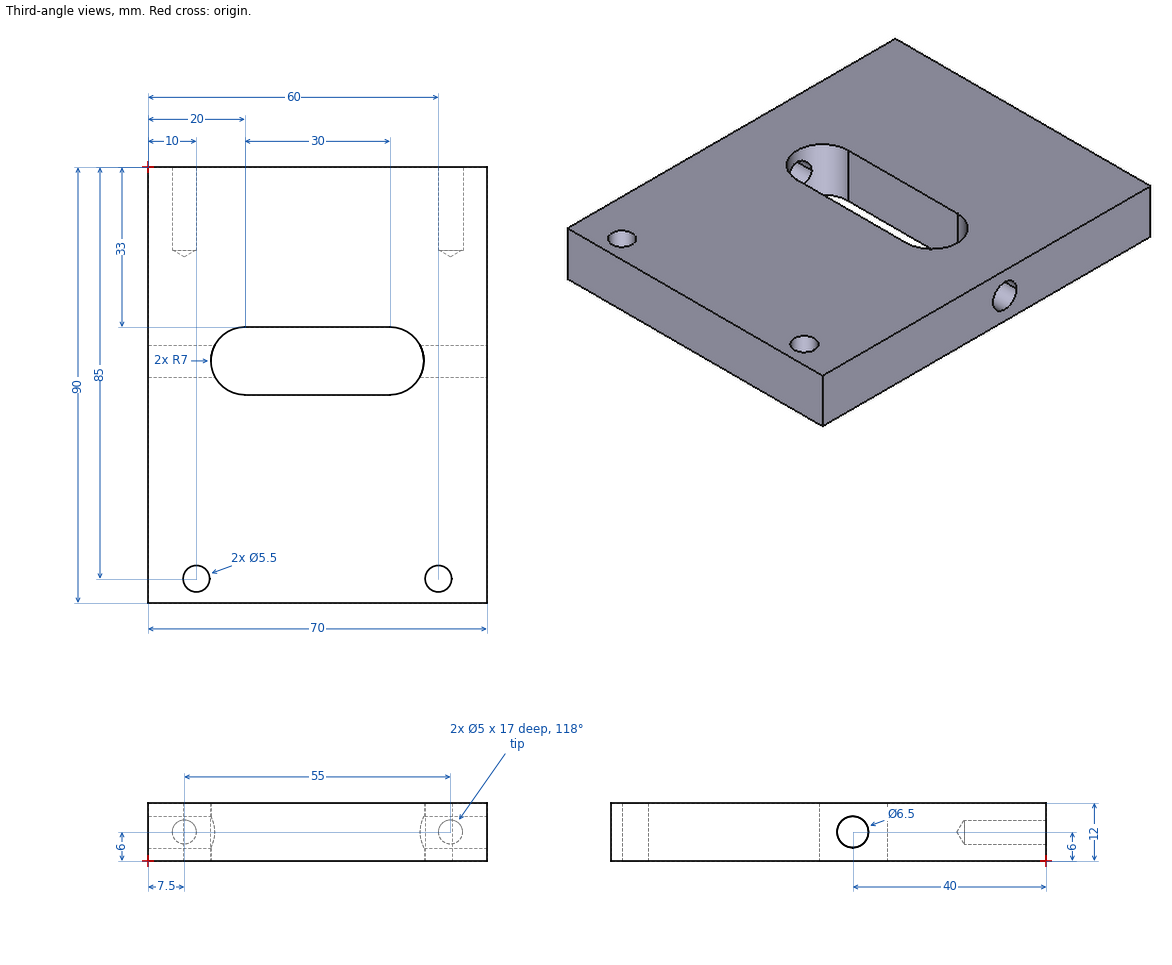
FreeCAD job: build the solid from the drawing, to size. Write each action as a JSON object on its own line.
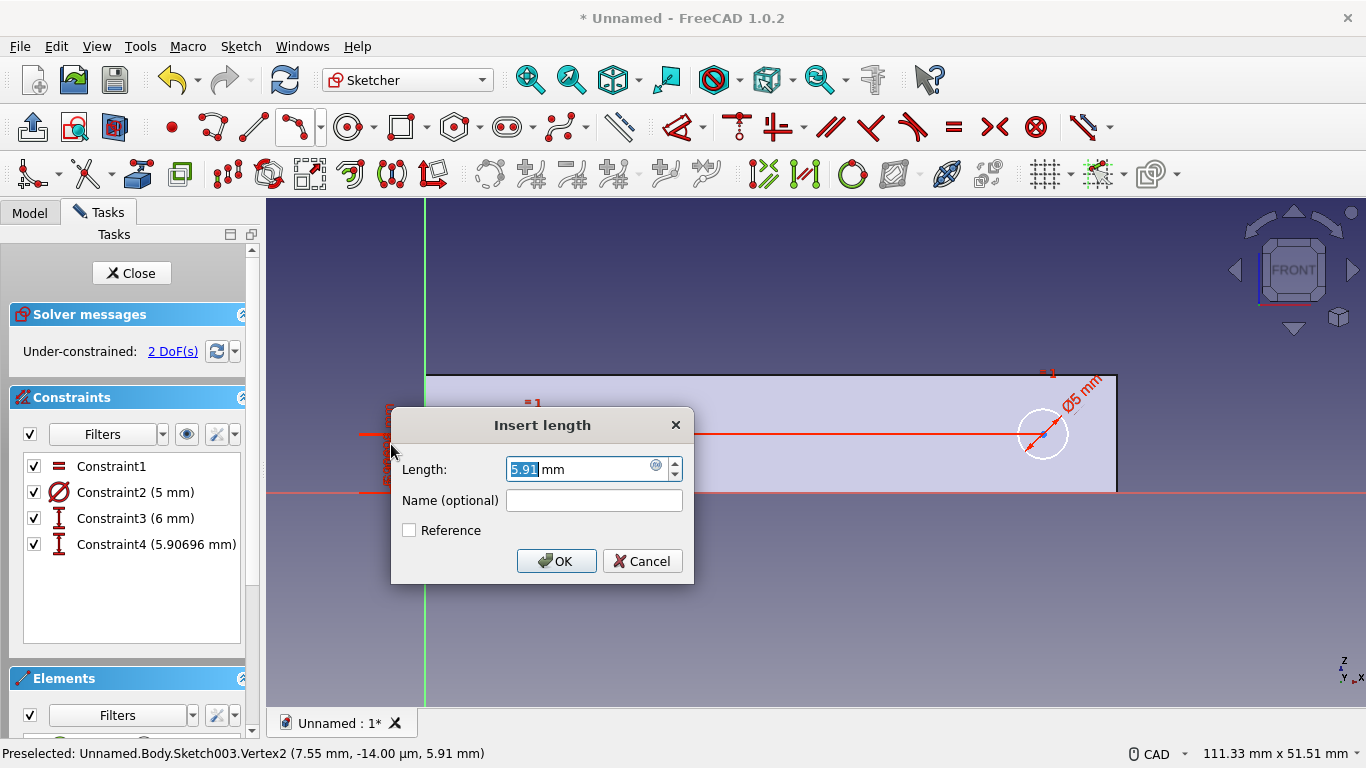
{"action": "type", "text": "6"}
{"action": "key", "text": "Return"}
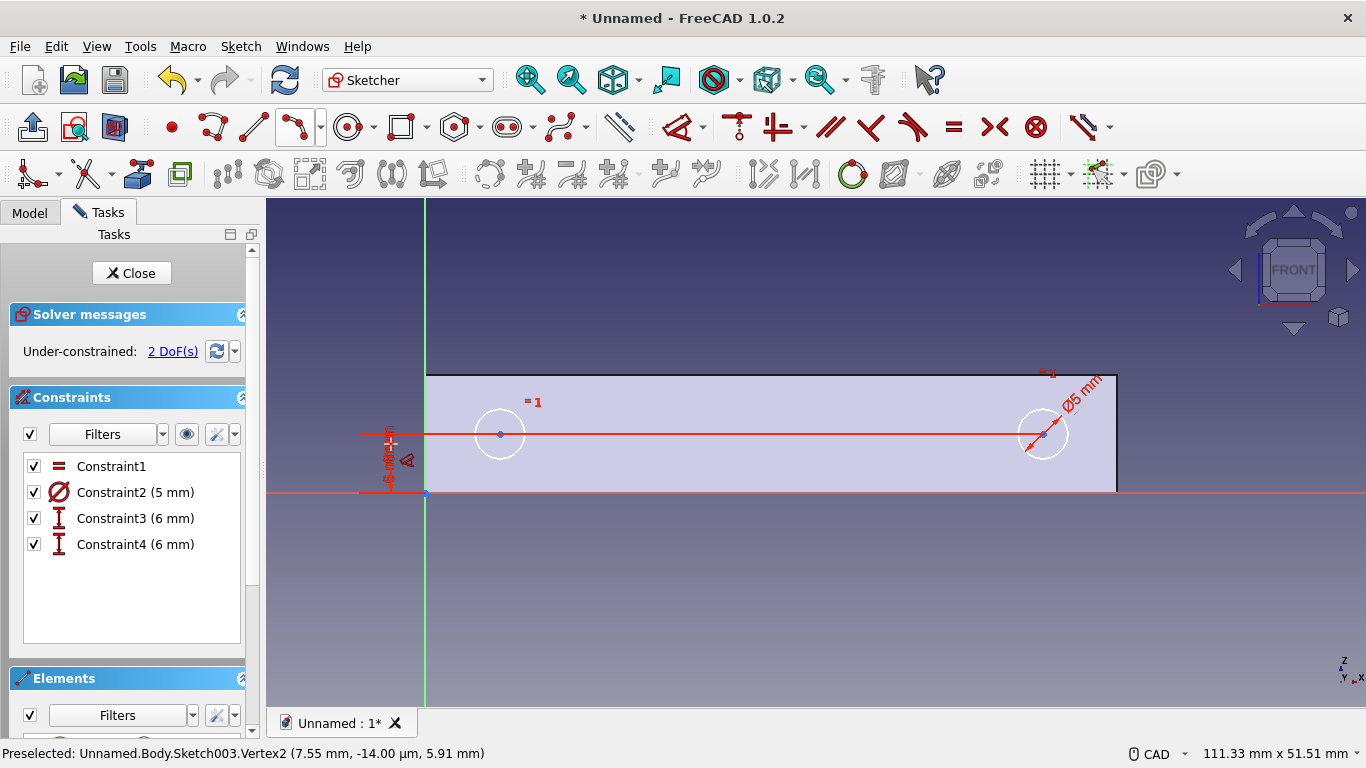
{"action": "left_click", "coordinate": [500, 434]}
{"action": "left_click", "coordinate": [463, 527]}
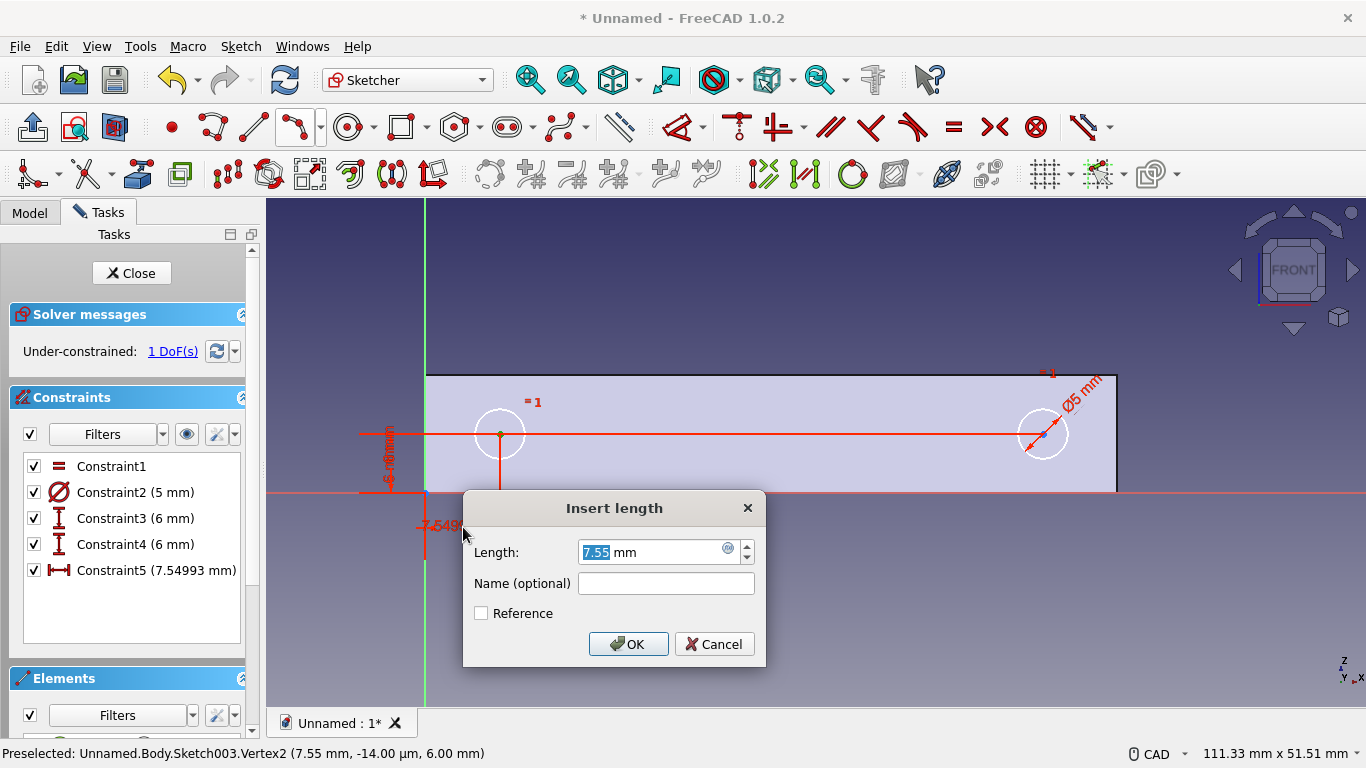
{"action": "type", "text": "7.5"}
{"action": "key", "text": "Return"}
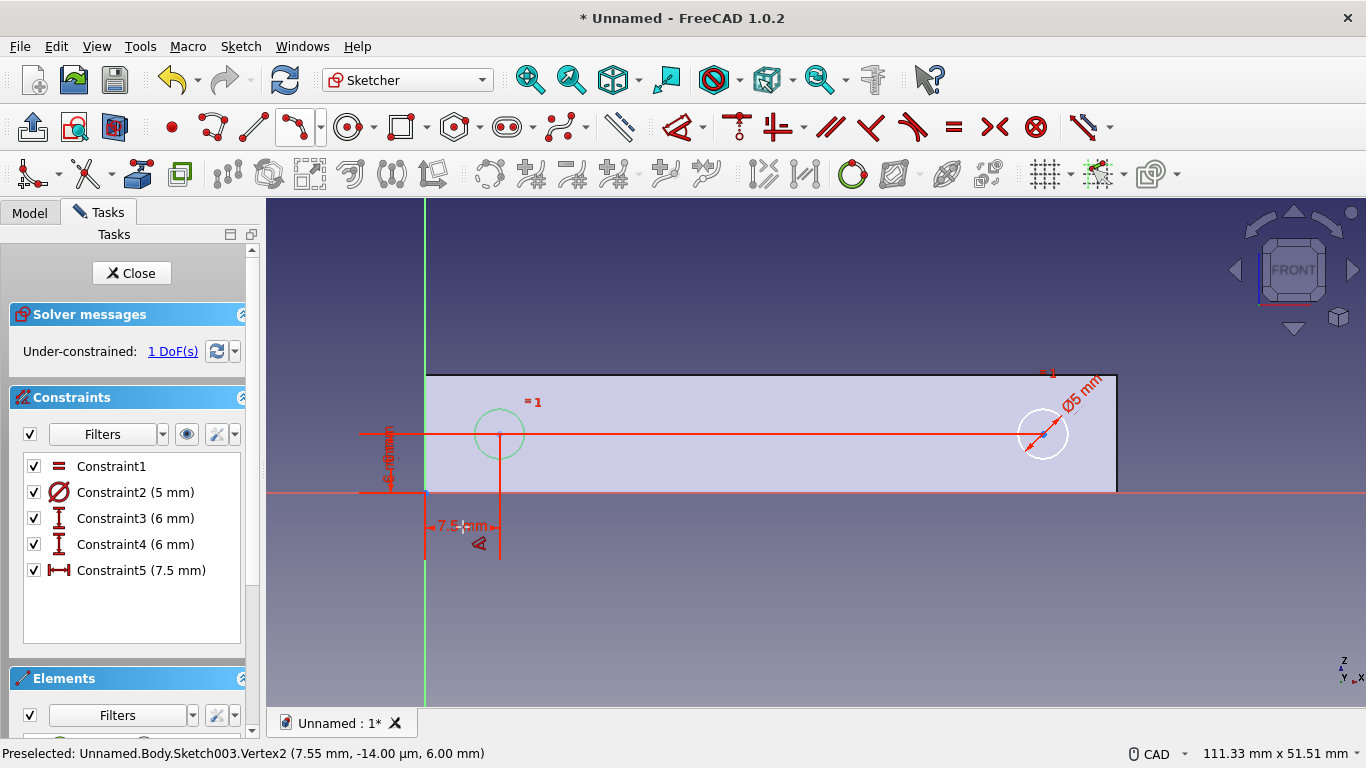
{"action": "left_click", "coordinate": [1043, 434]}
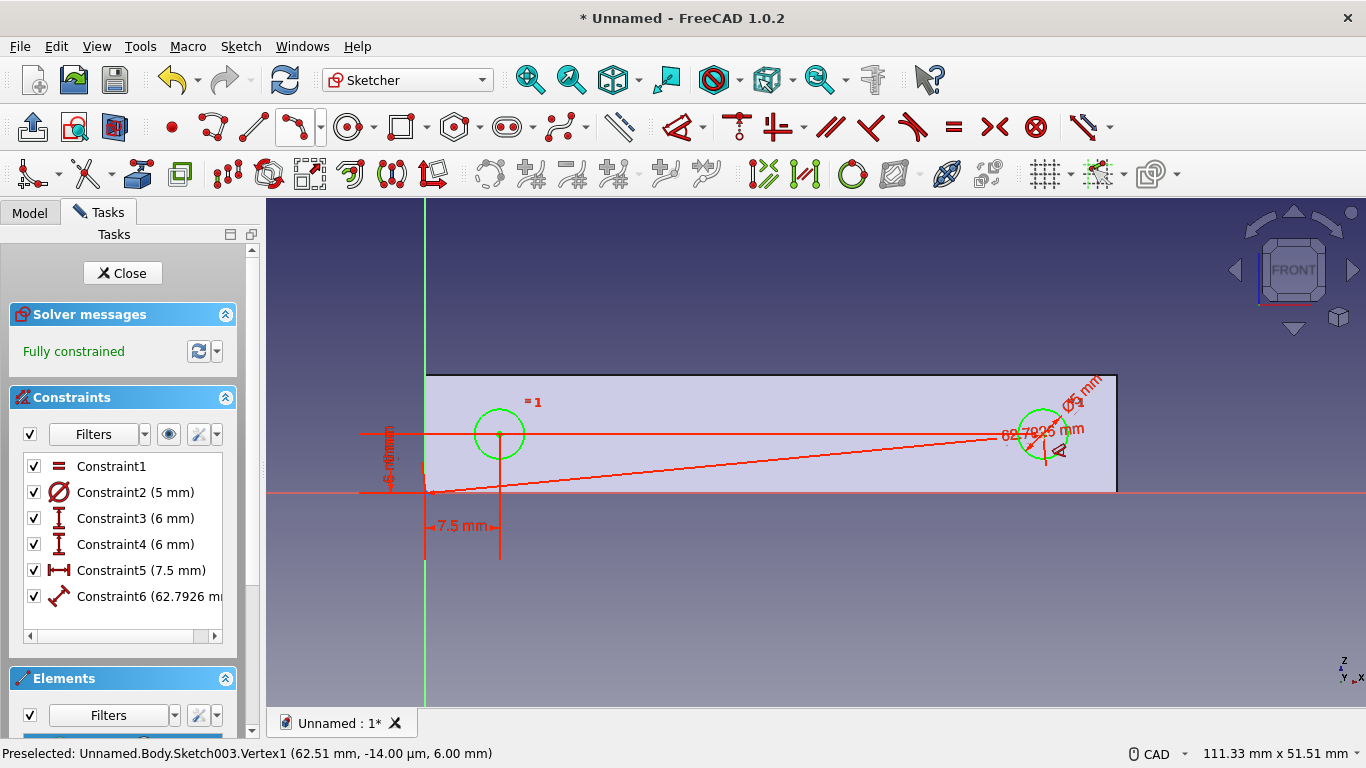
{"action": "left_click", "coordinate": [500, 434]}
{"action": "left_click", "coordinate": [771, 400]}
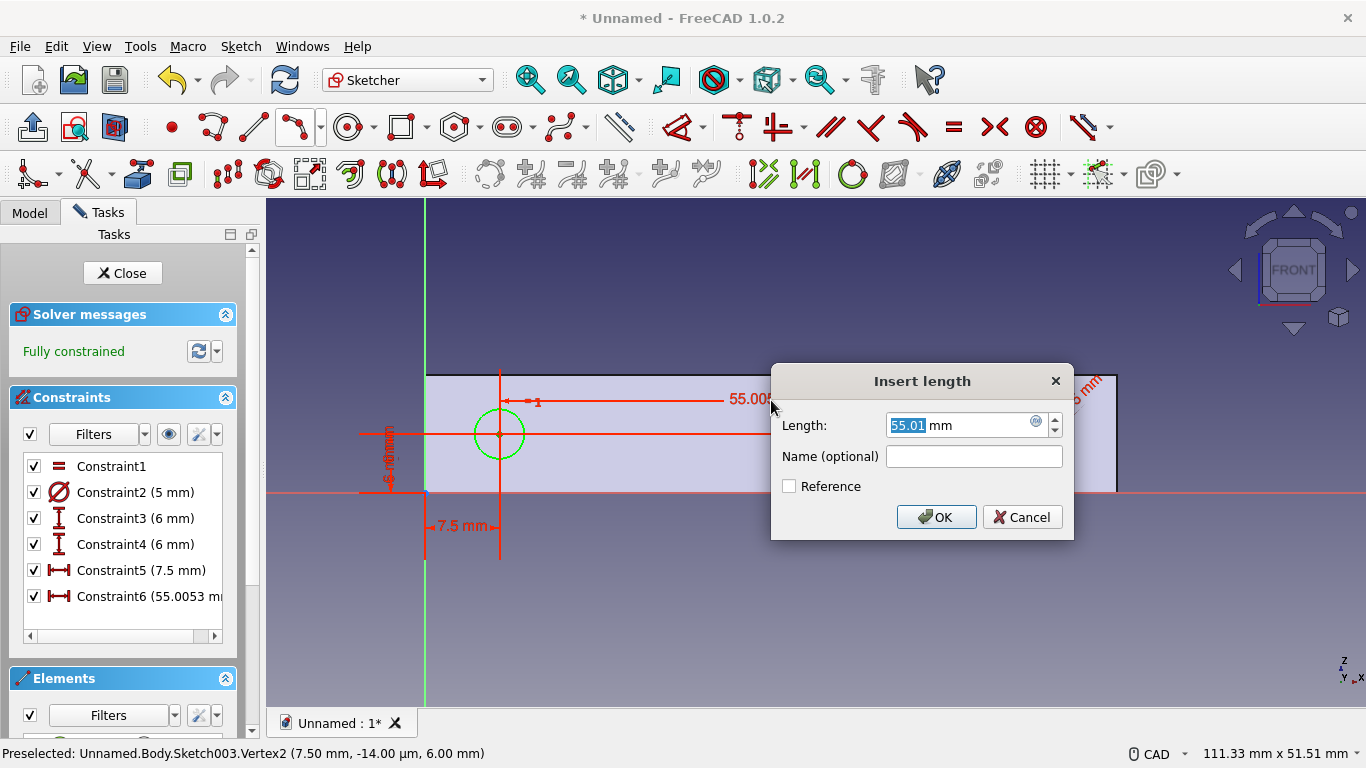
{"action": "type", "text": "55"}
{"action": "key", "text": "Return"}
{"action": "key", "text": "Escape"}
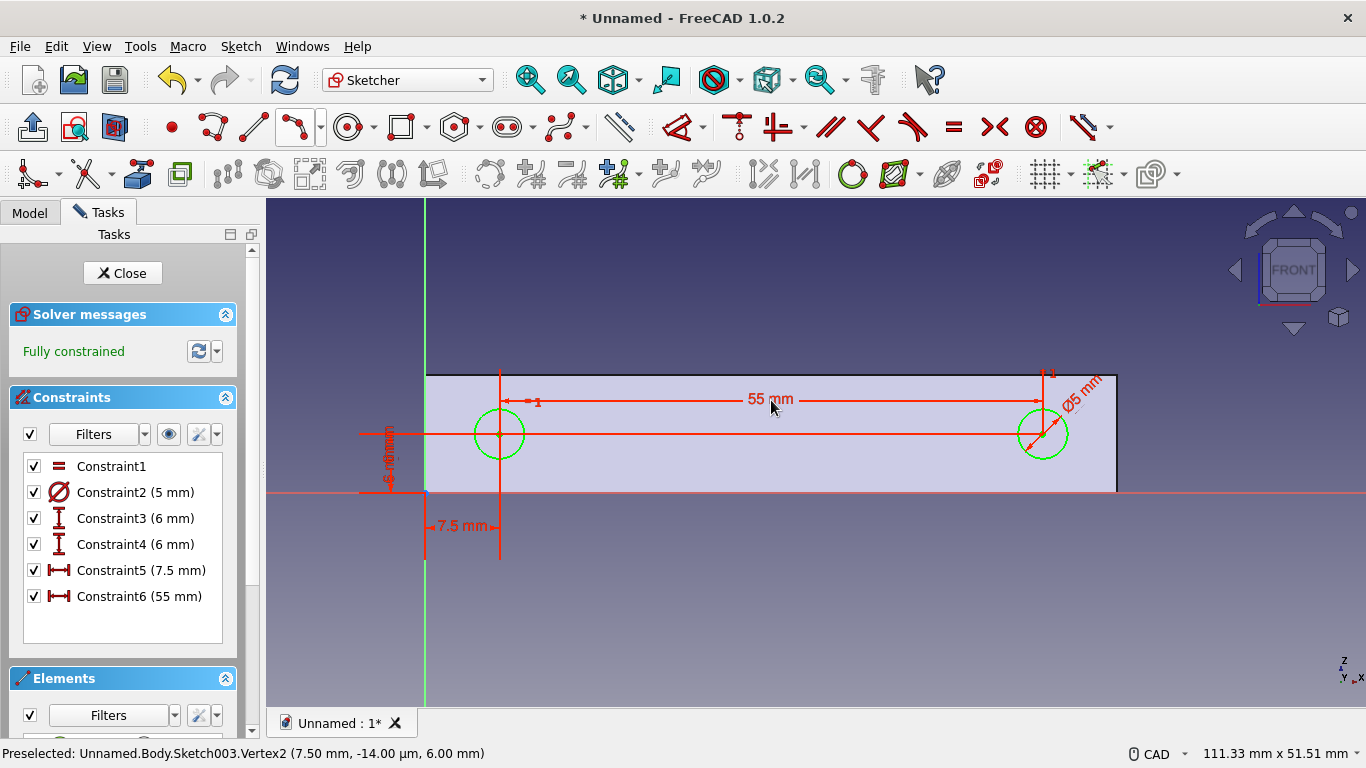
{"action": "left_click", "coordinate": [123, 273]}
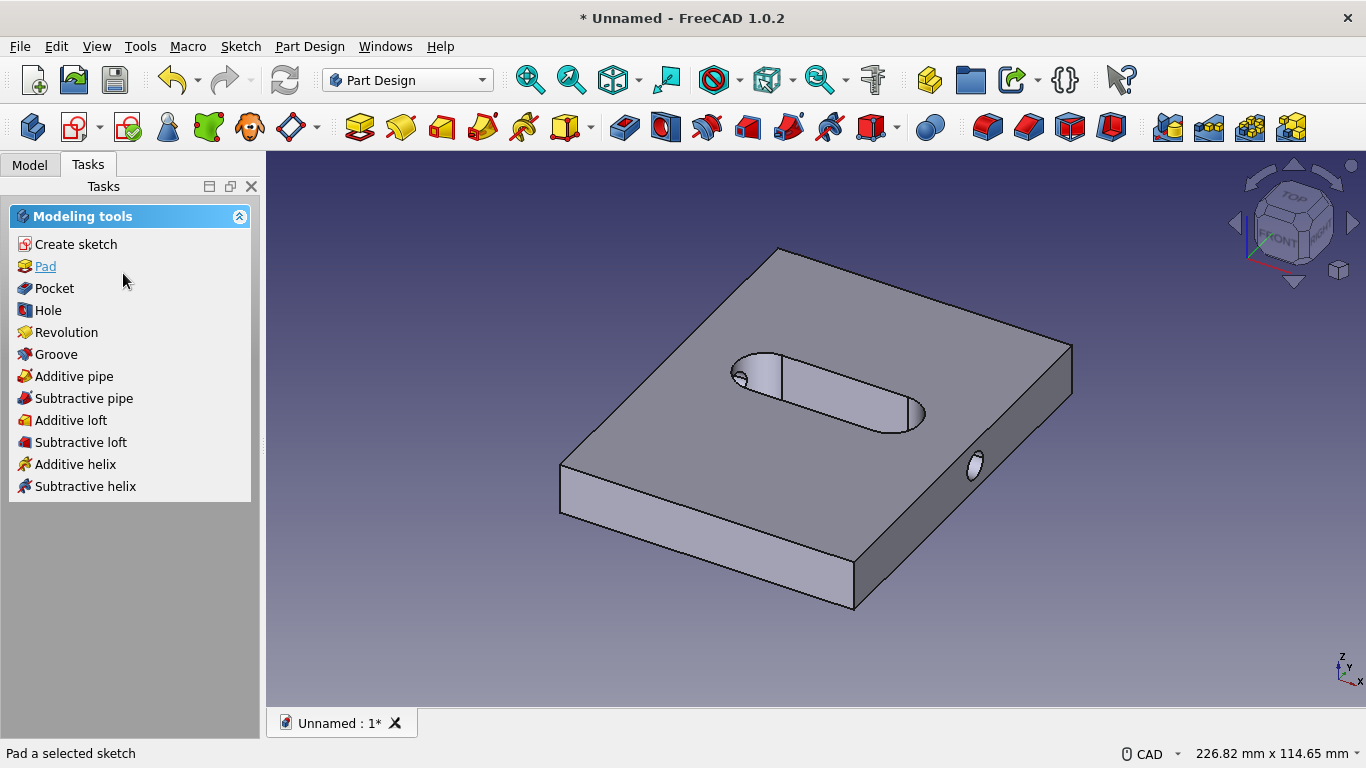
{"action": "left_click", "coordinate": [666, 128]}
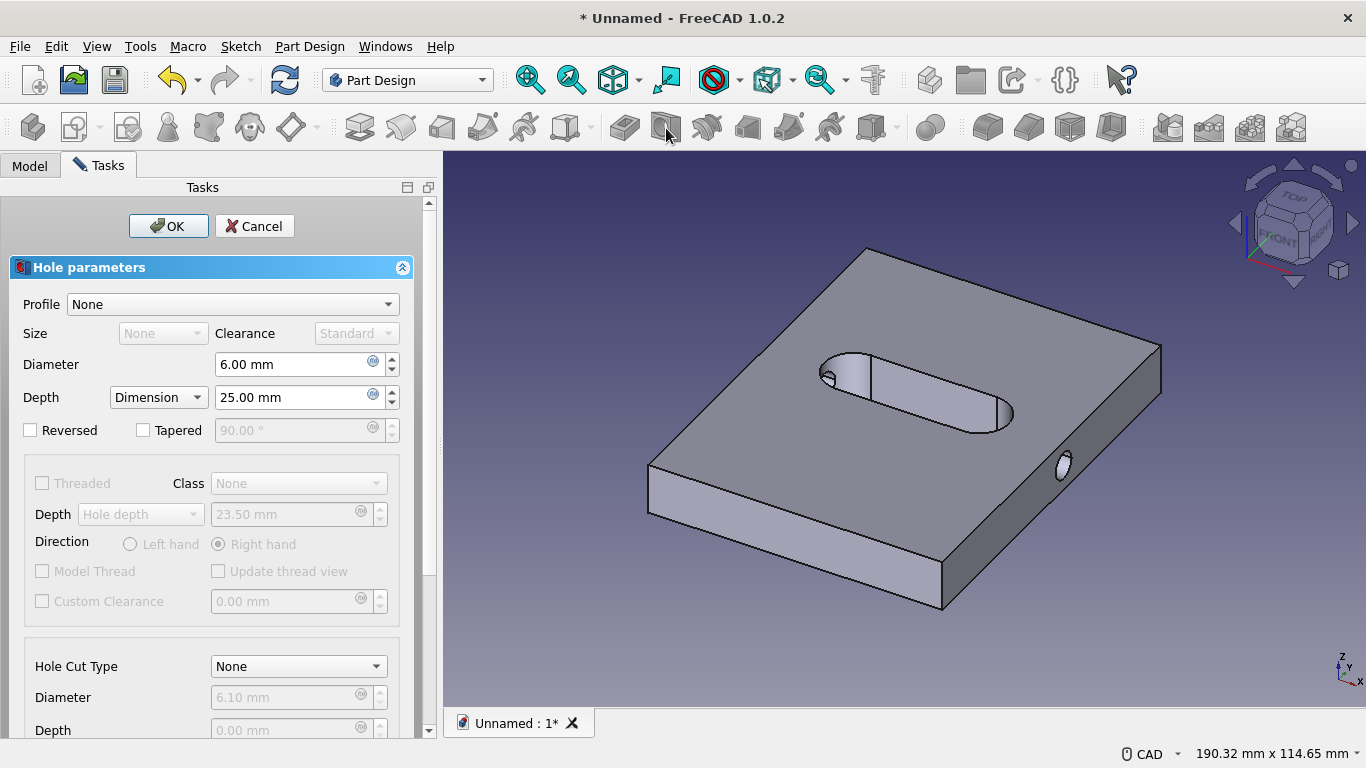
{"action": "triple_click", "coordinate": [300, 364]}